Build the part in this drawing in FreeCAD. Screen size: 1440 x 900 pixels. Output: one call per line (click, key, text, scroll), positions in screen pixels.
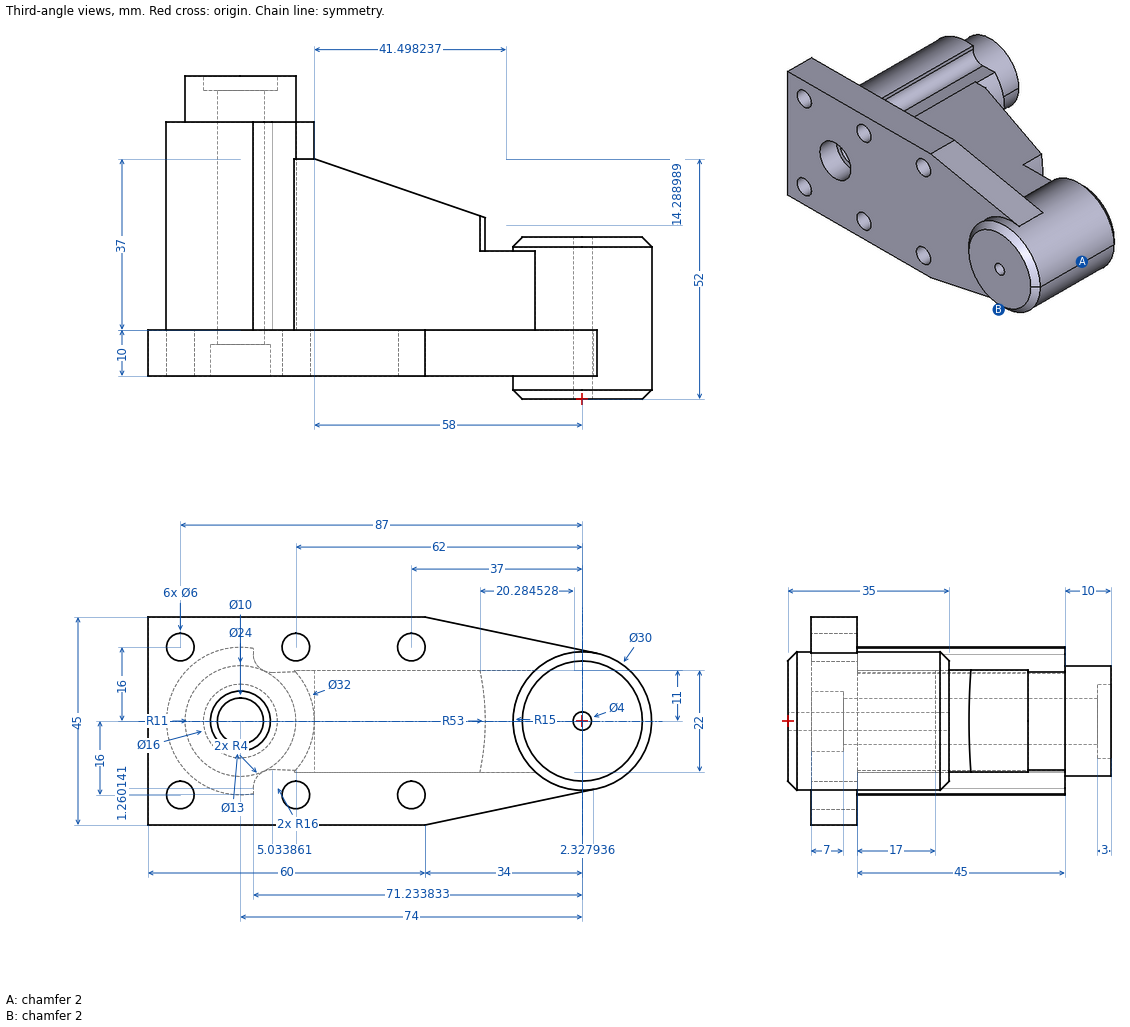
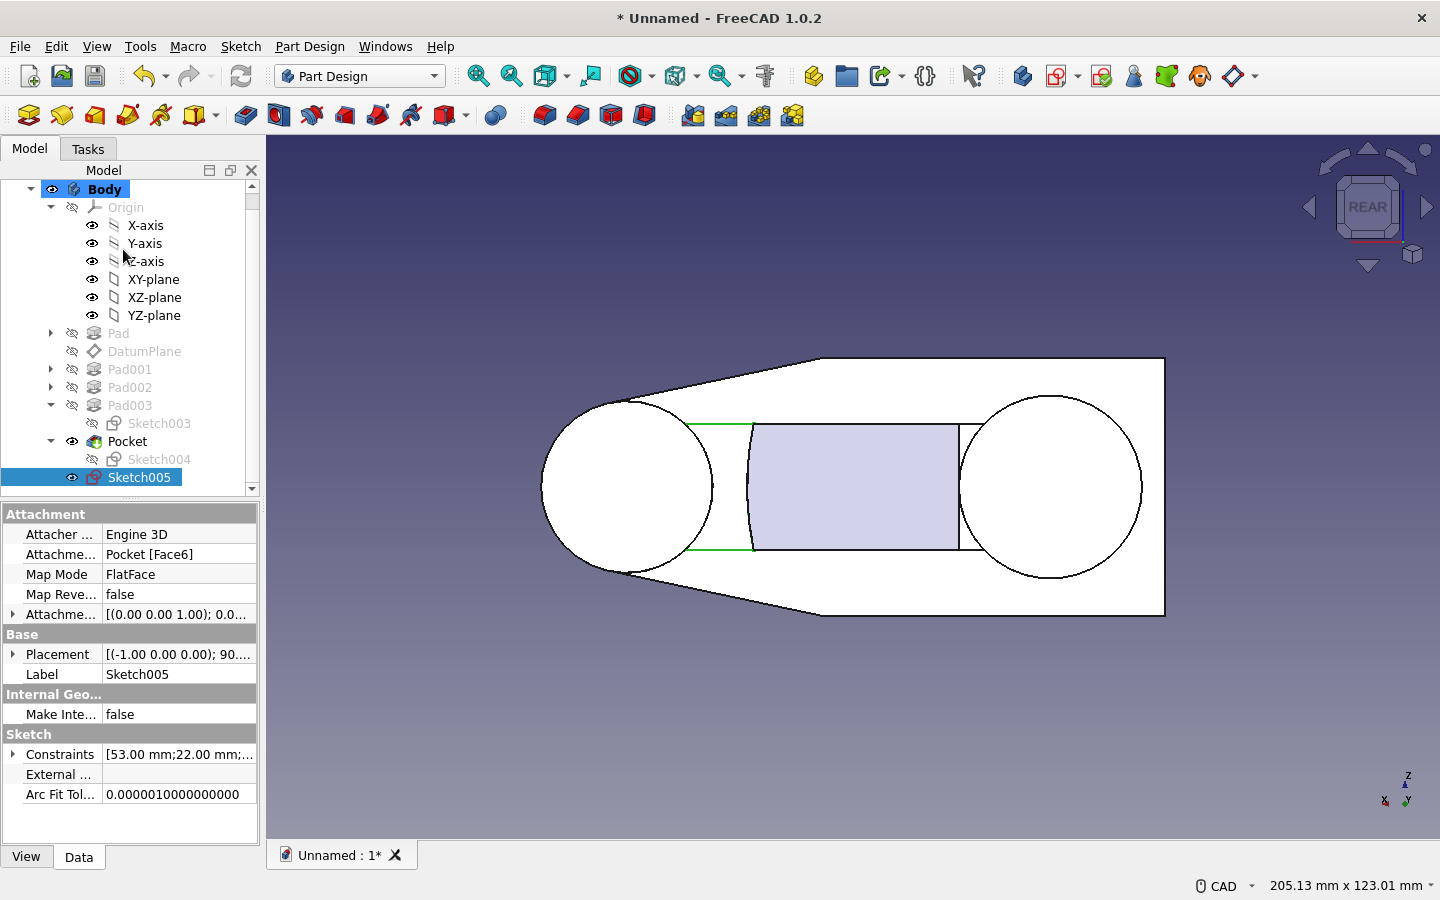
click(29, 116)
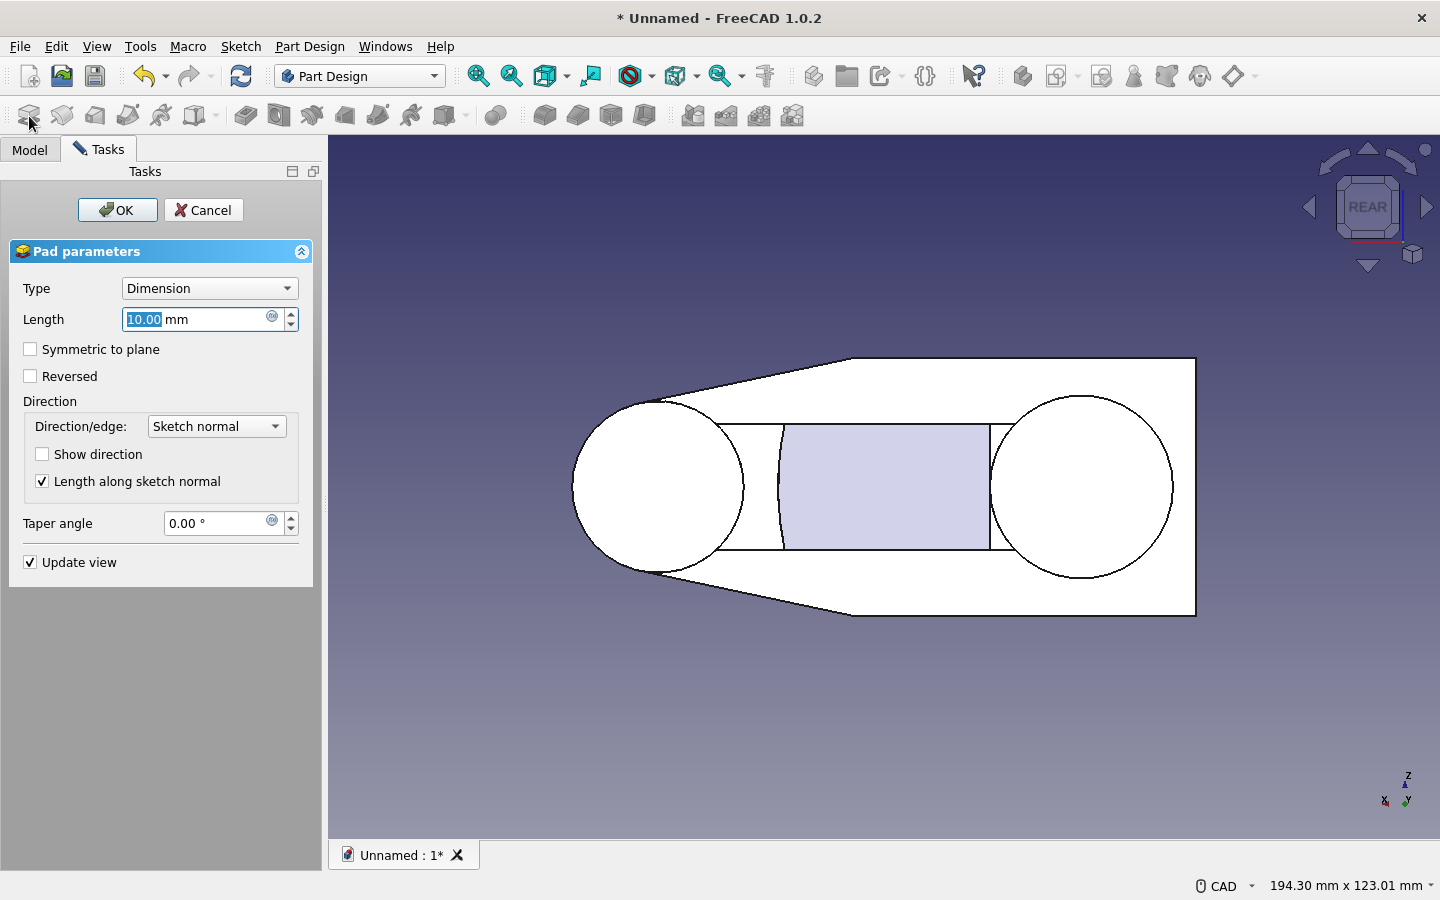
text(17)
key(Tab)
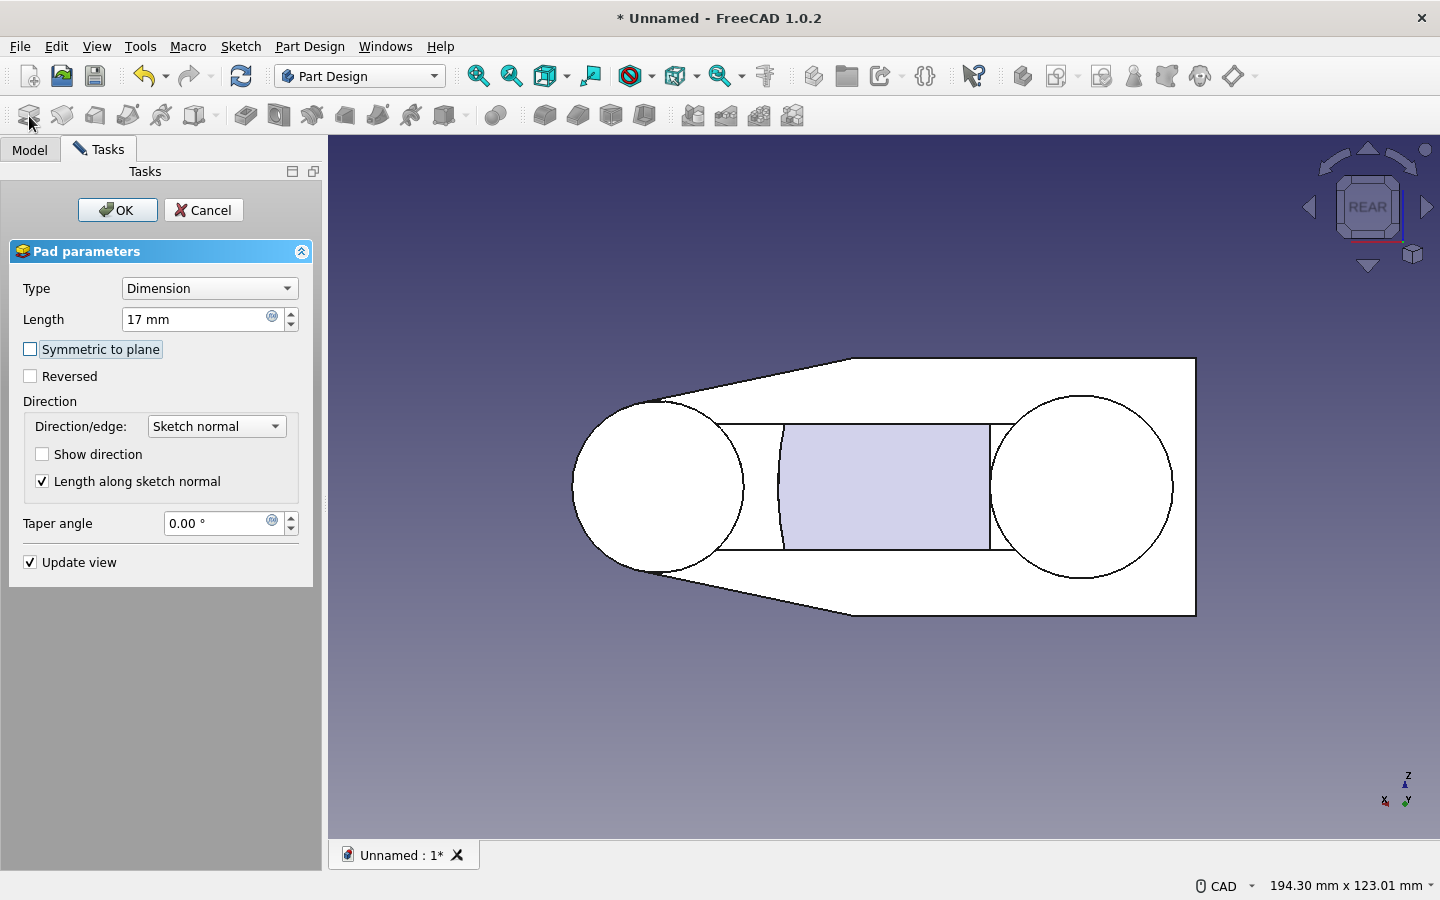
click(118, 210)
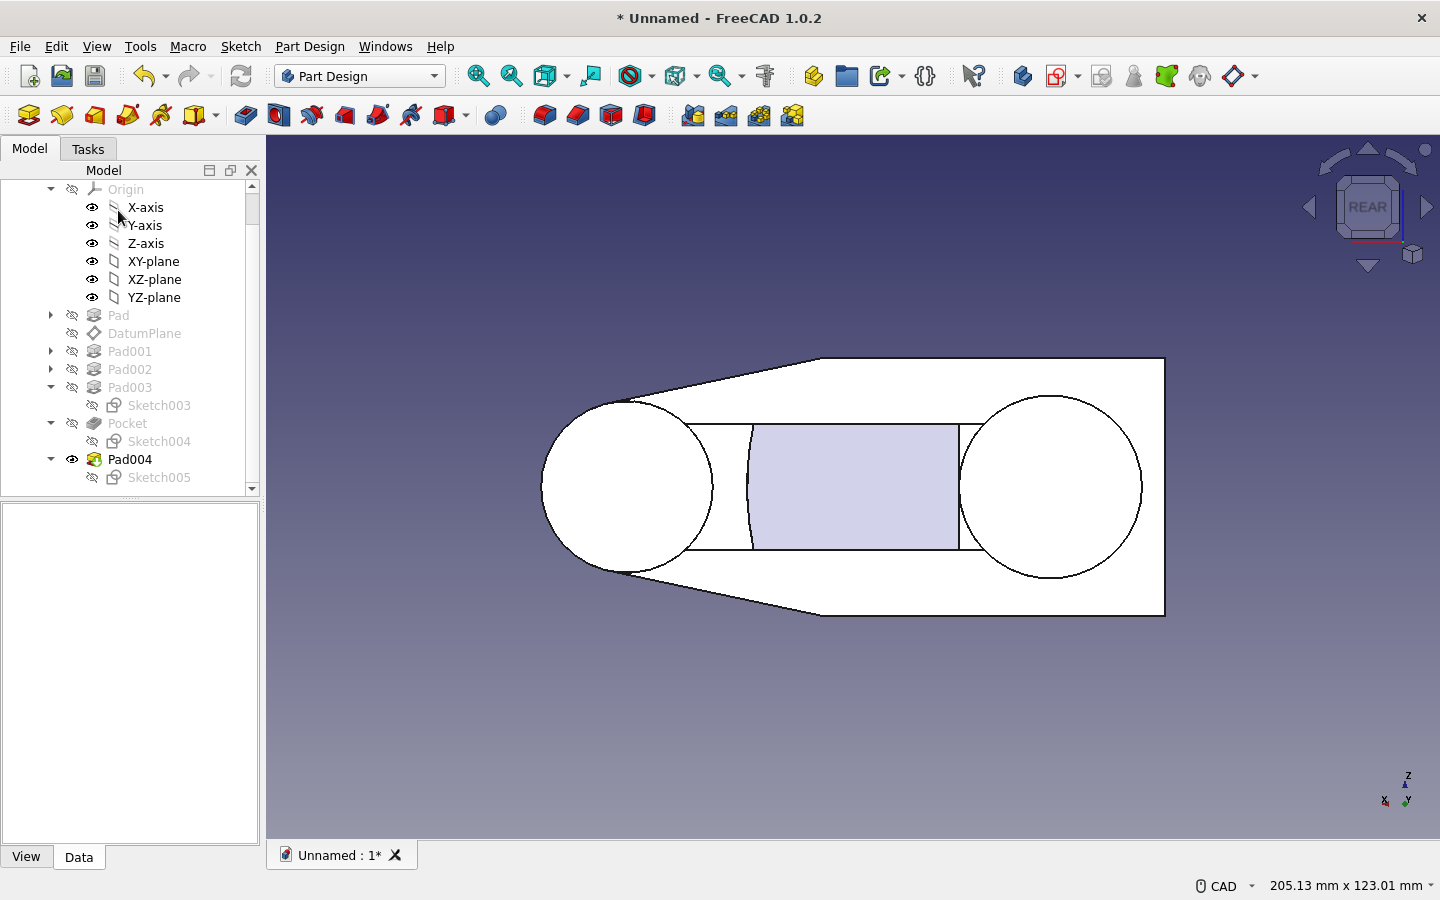
click(713, 486)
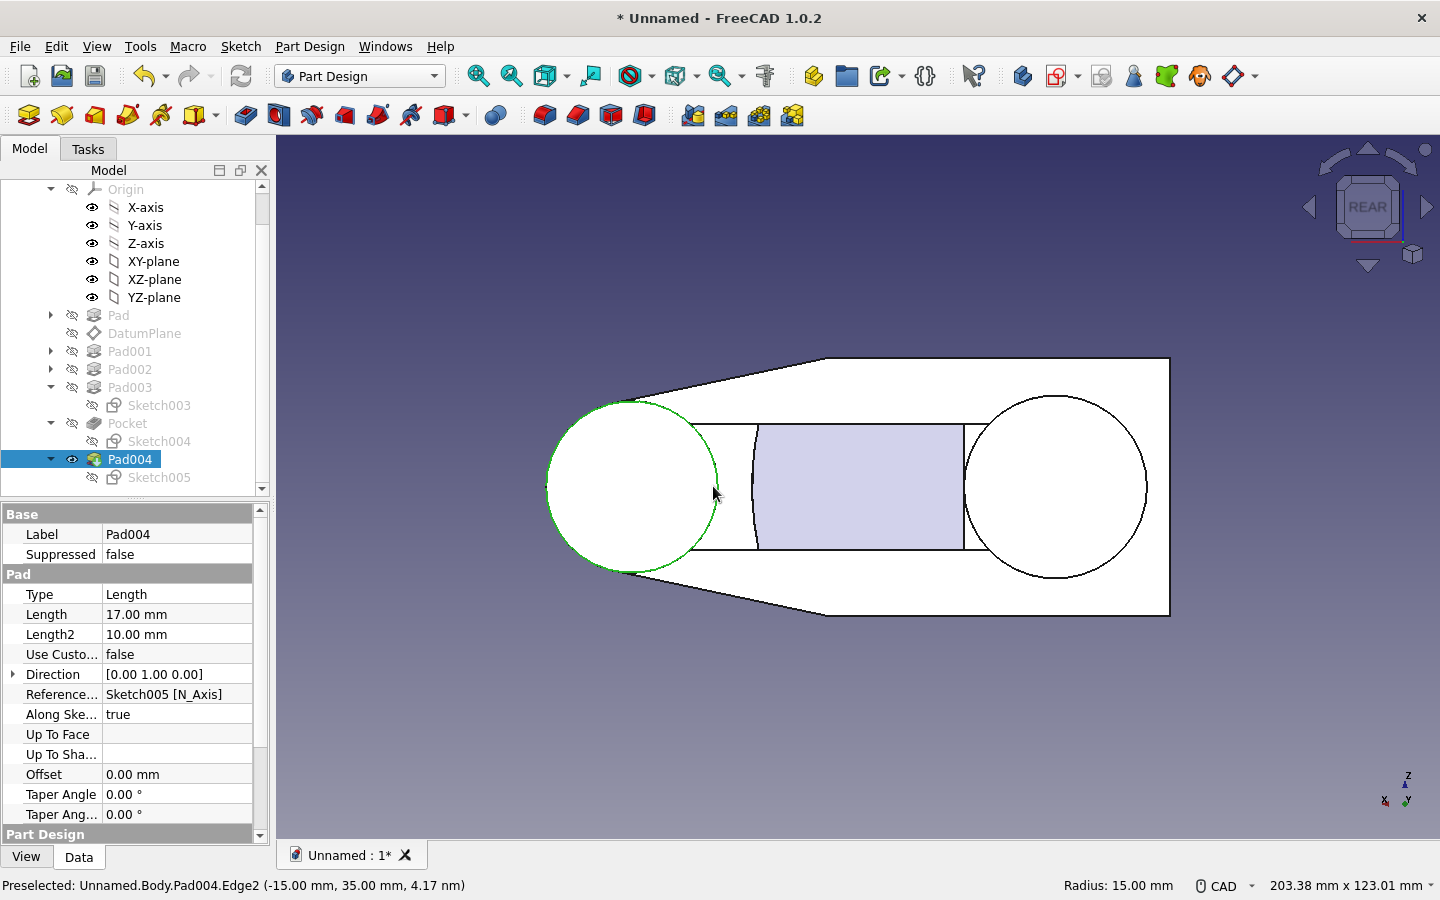
click(578, 116)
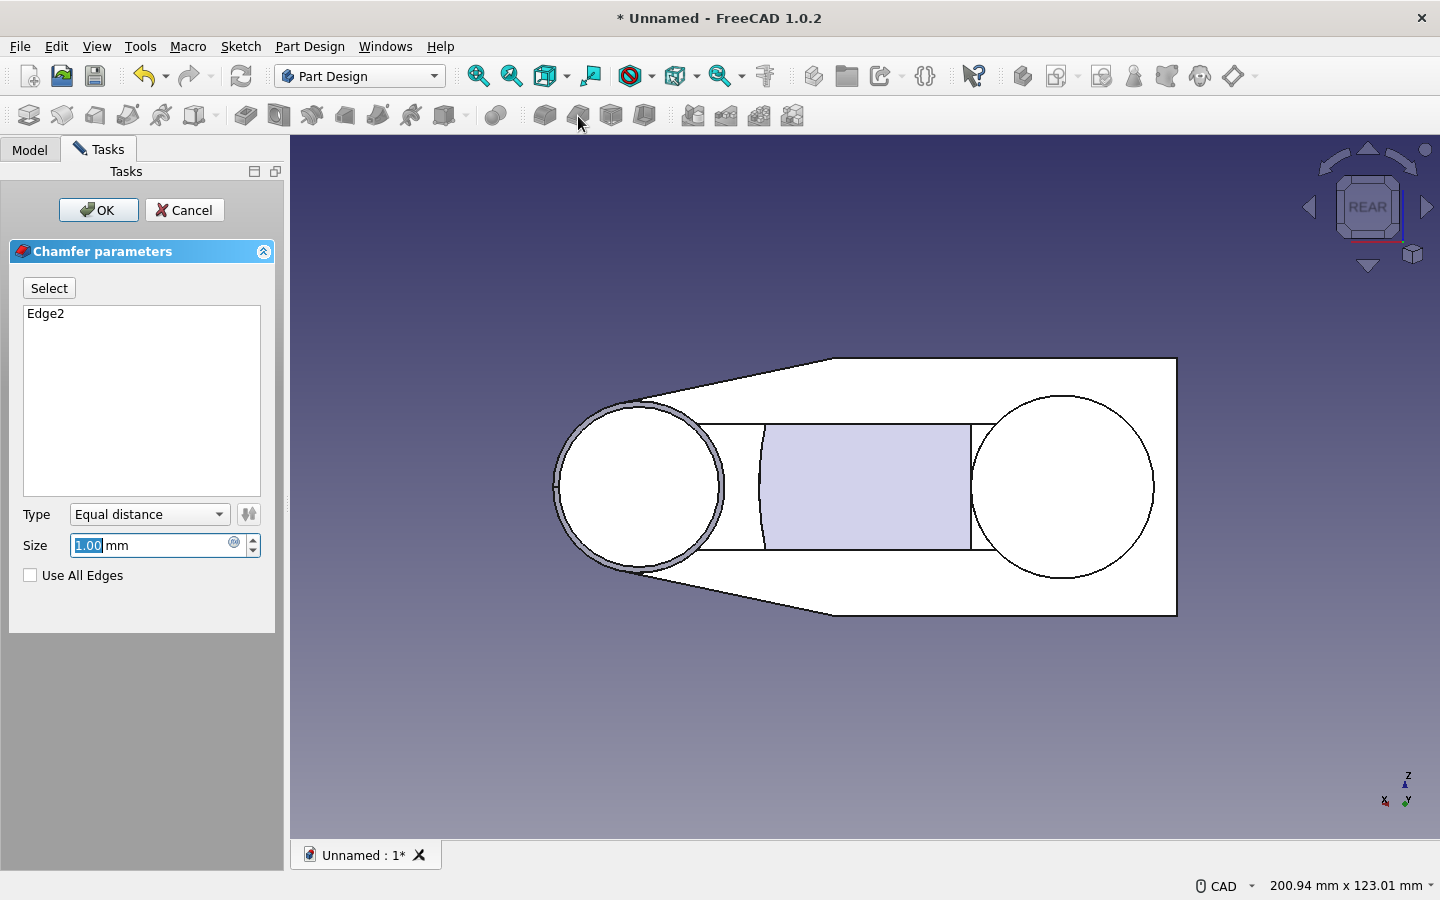
text(2)
key(Tab)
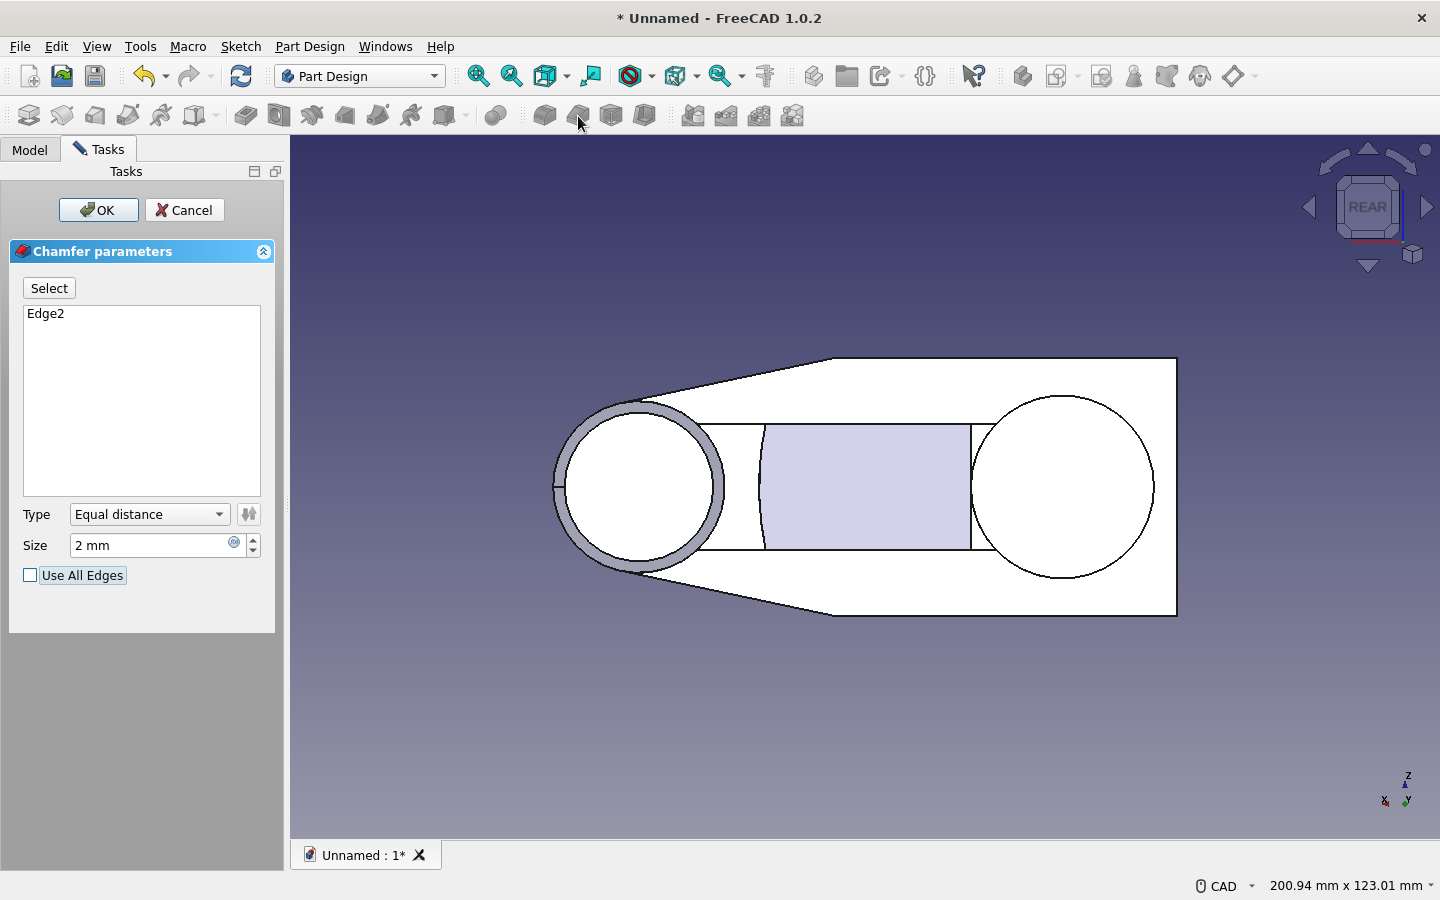
click(99, 210)